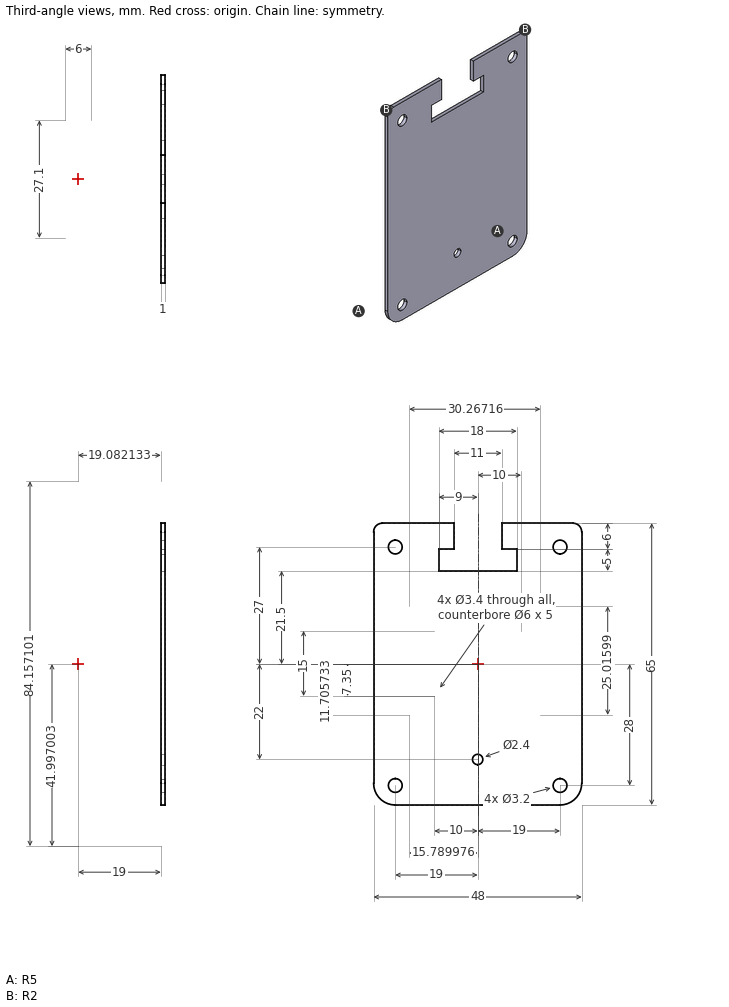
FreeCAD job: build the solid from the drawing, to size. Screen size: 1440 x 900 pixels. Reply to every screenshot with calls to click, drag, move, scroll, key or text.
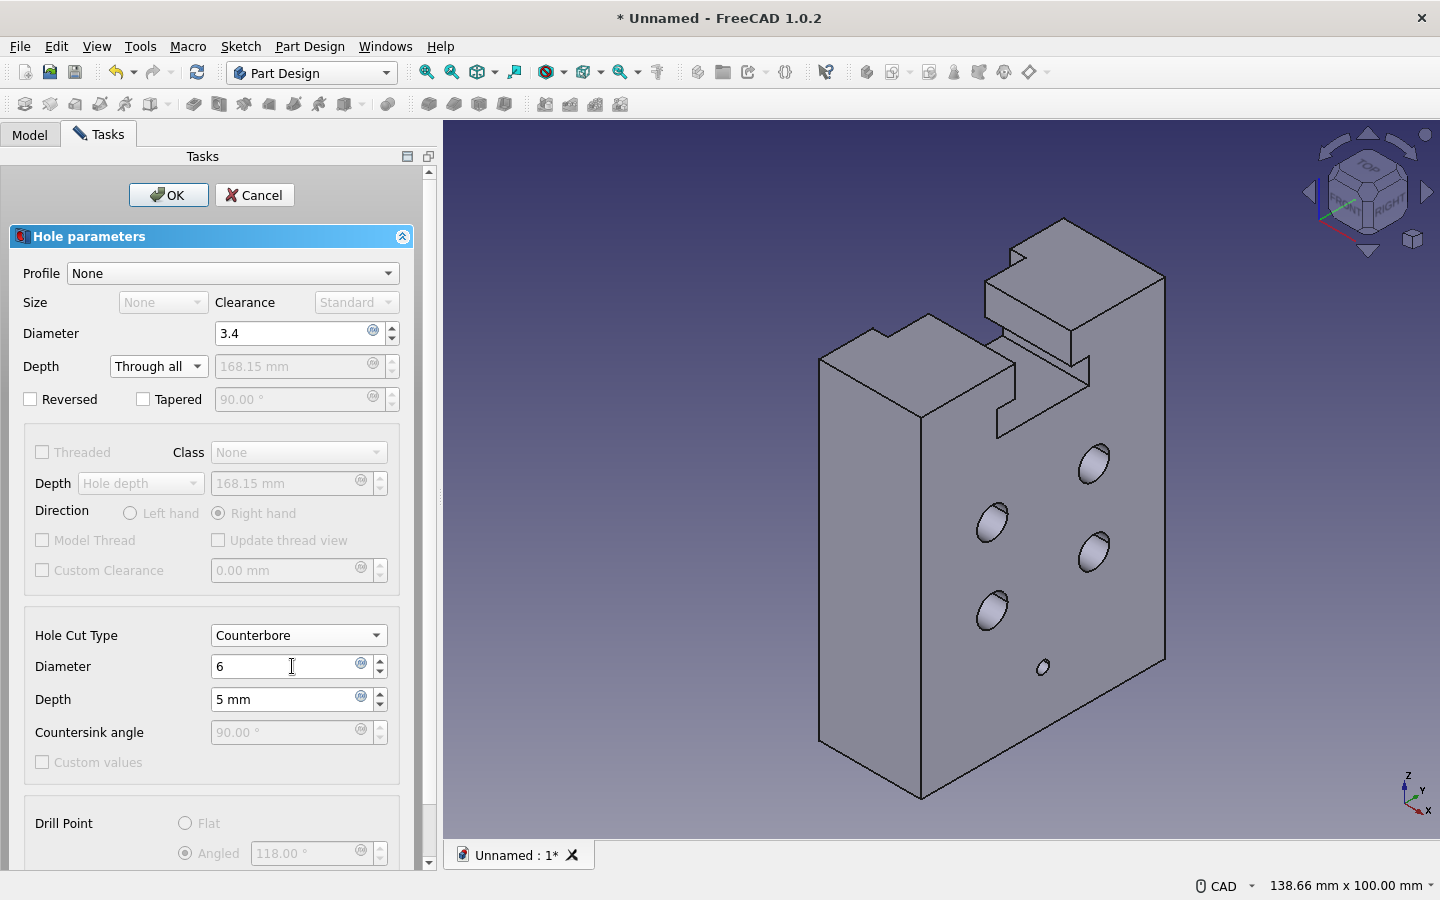
click(169, 195)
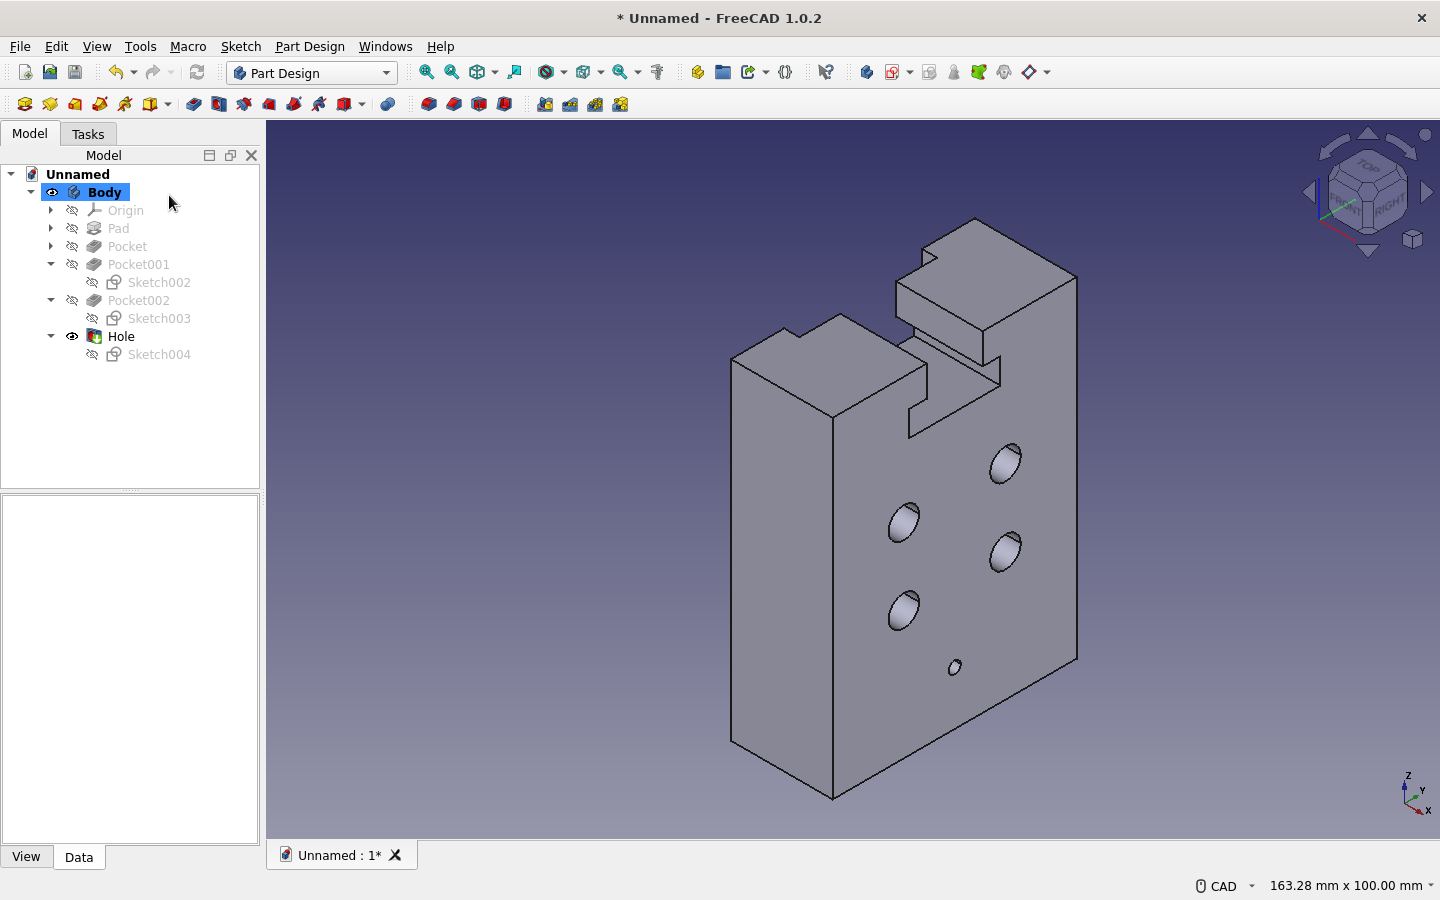
key(2)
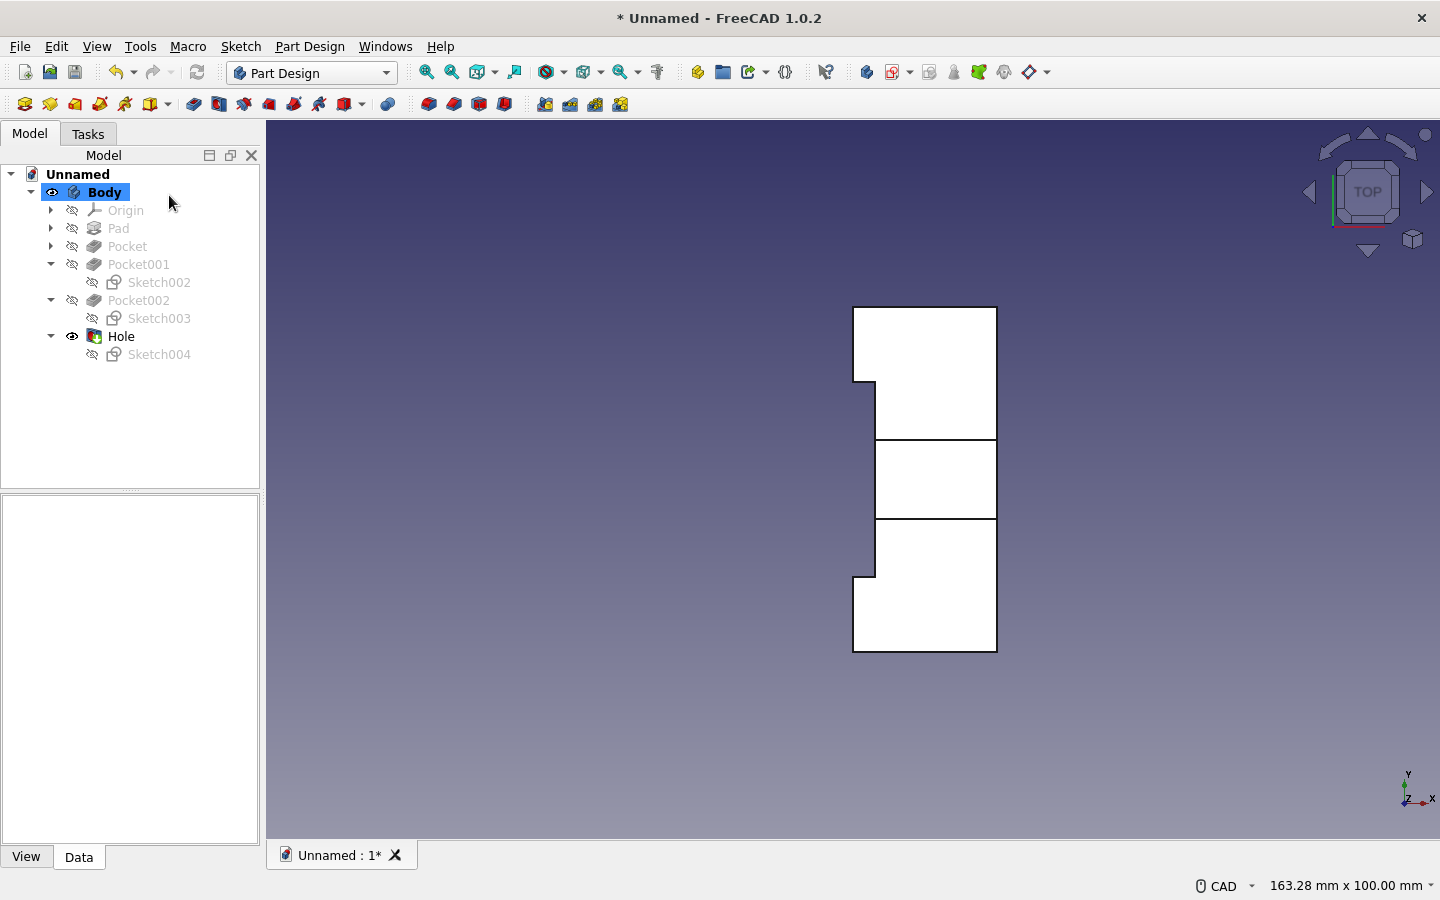
key(0)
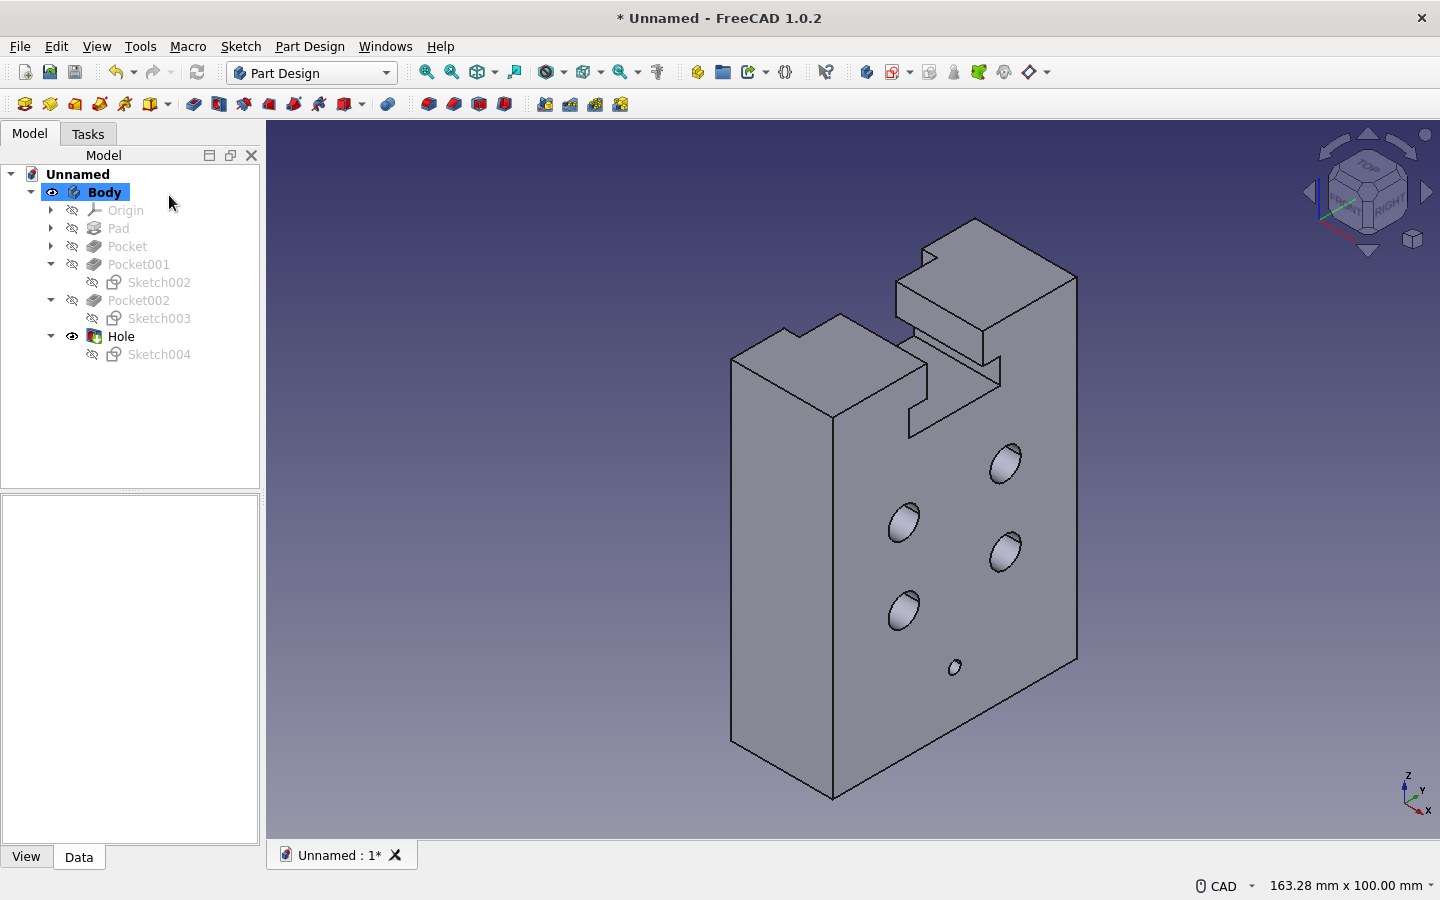
key(1)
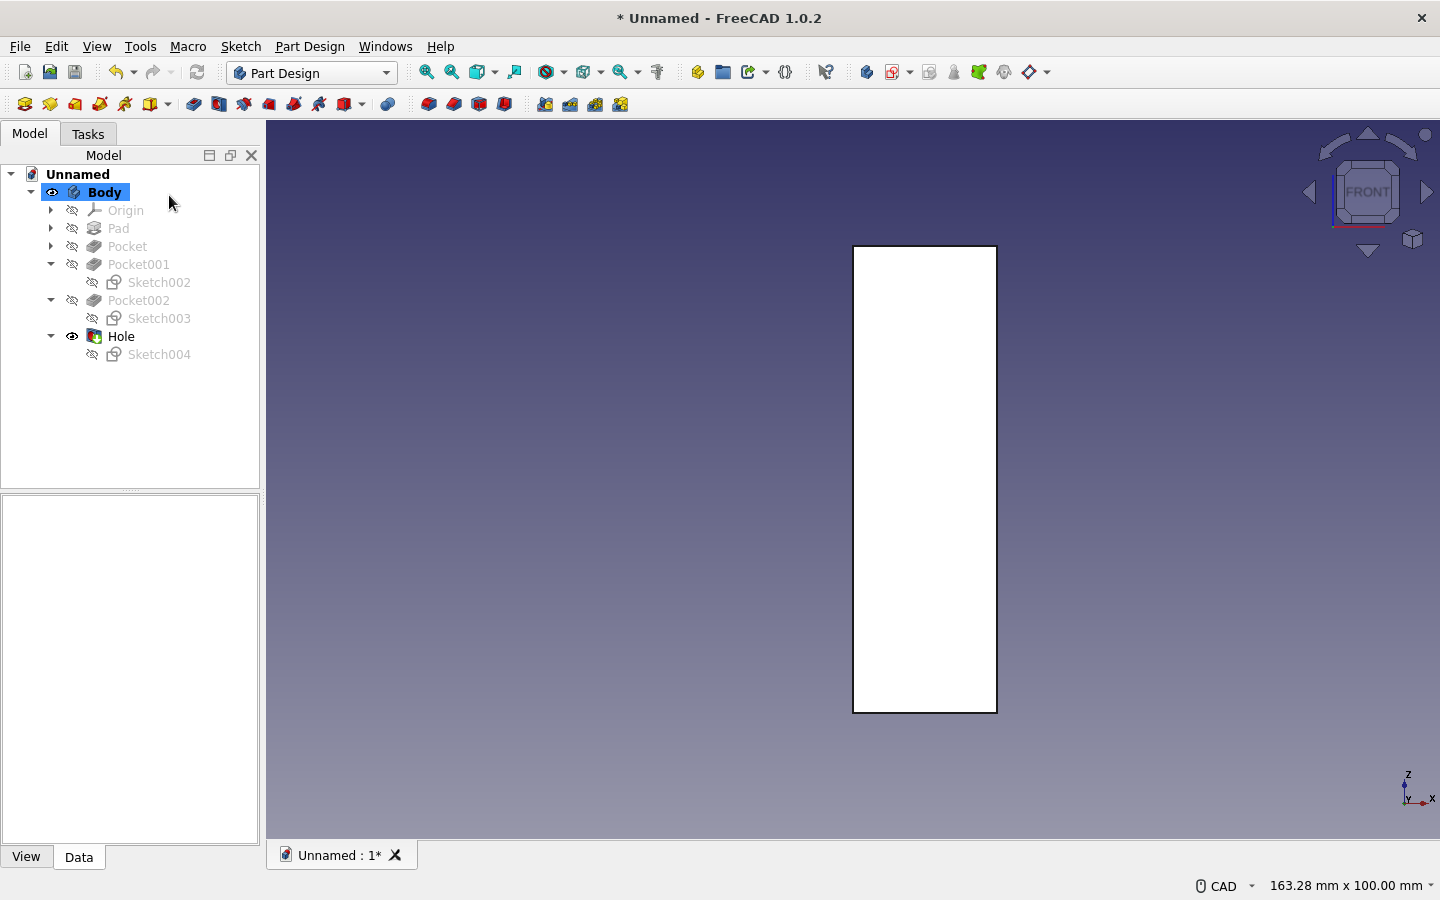
click(925, 712)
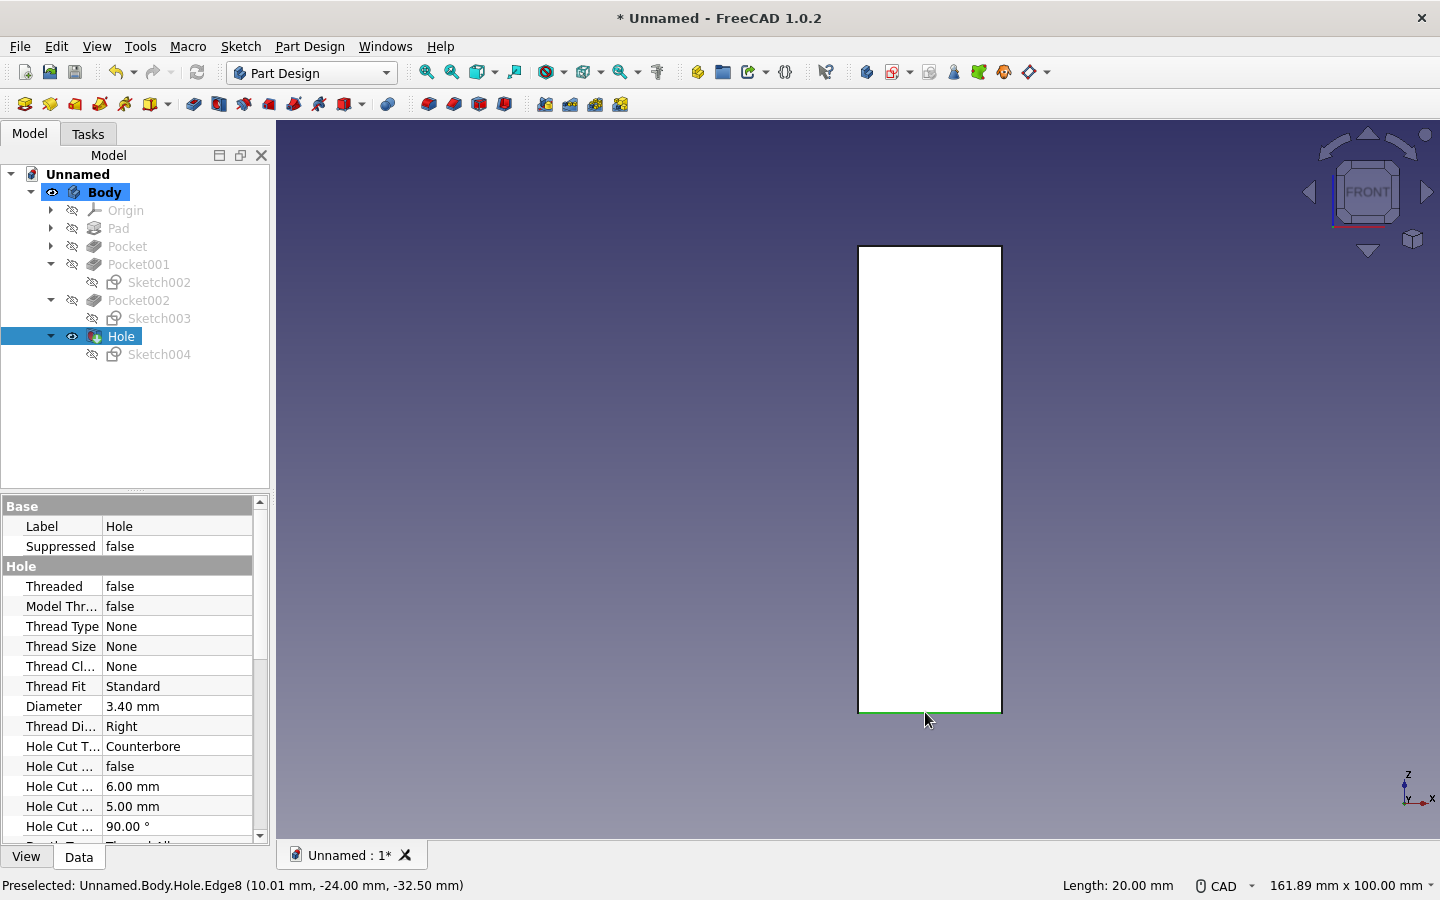
key(3)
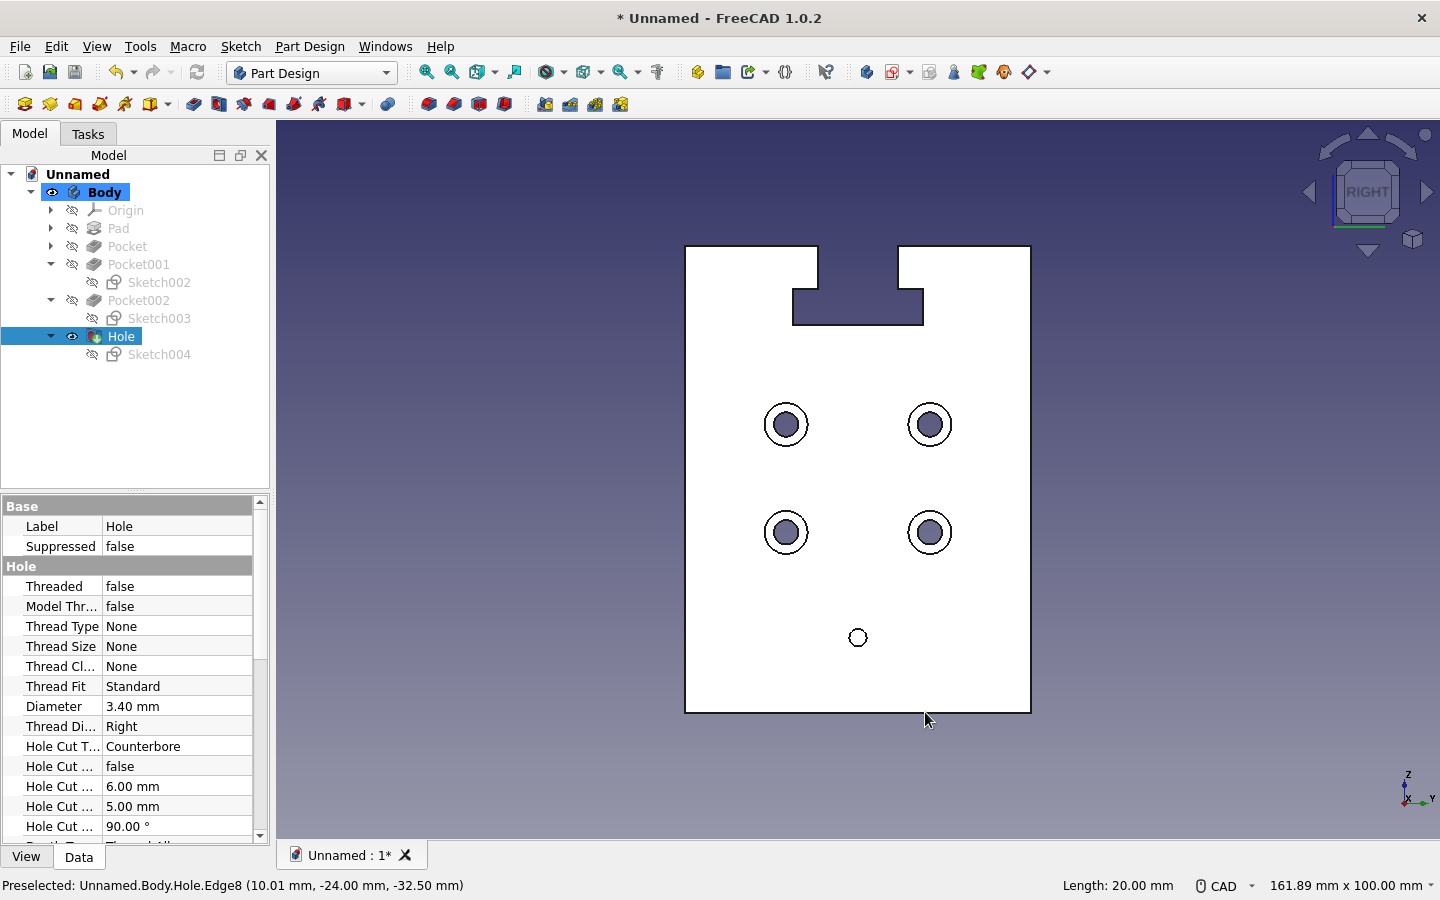
key(5)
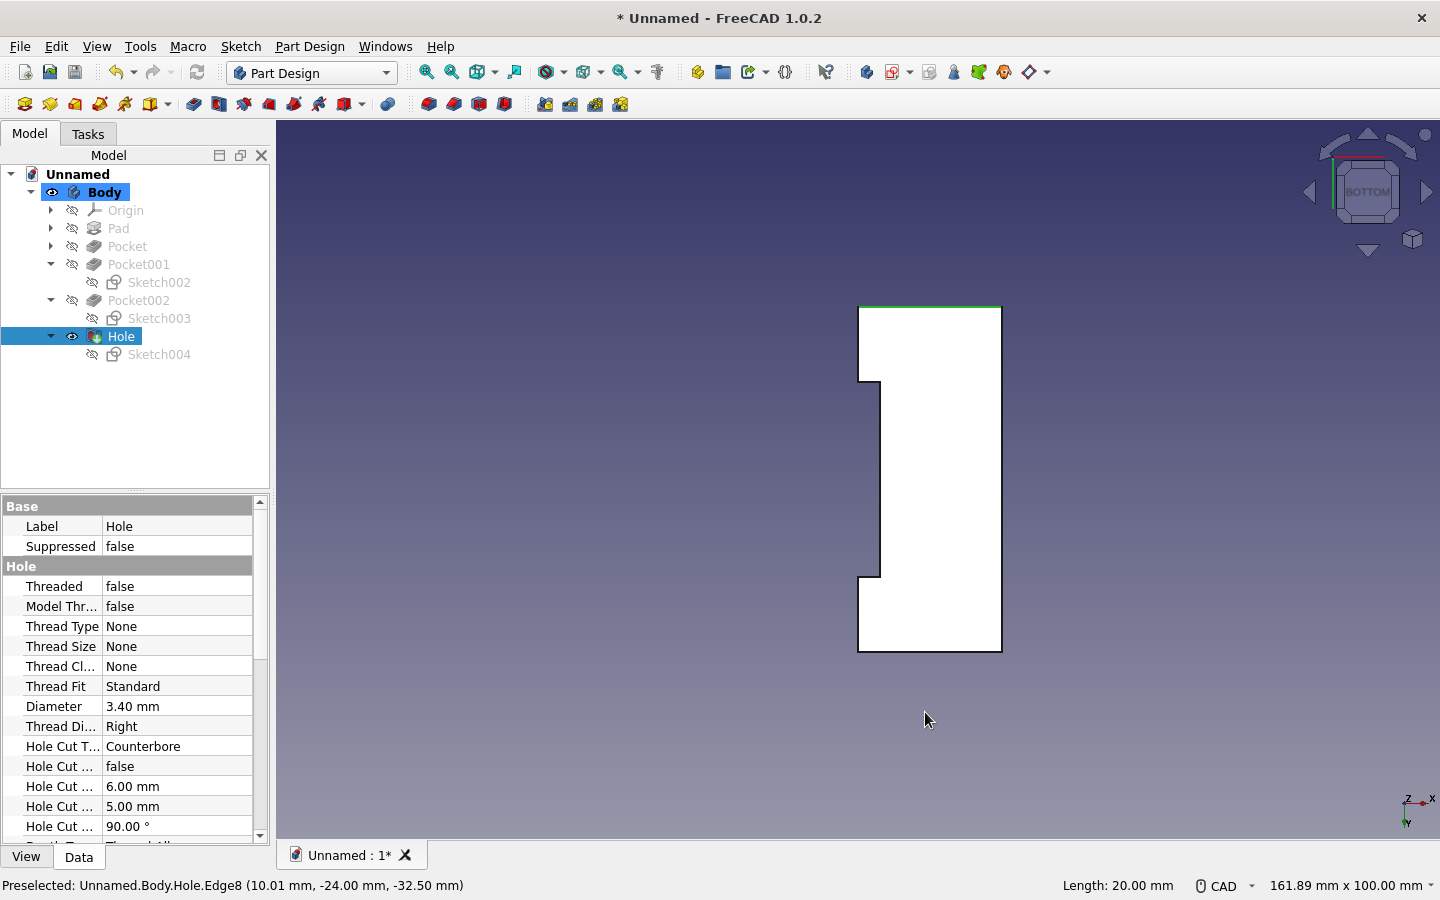
click(930, 651, ctrl)